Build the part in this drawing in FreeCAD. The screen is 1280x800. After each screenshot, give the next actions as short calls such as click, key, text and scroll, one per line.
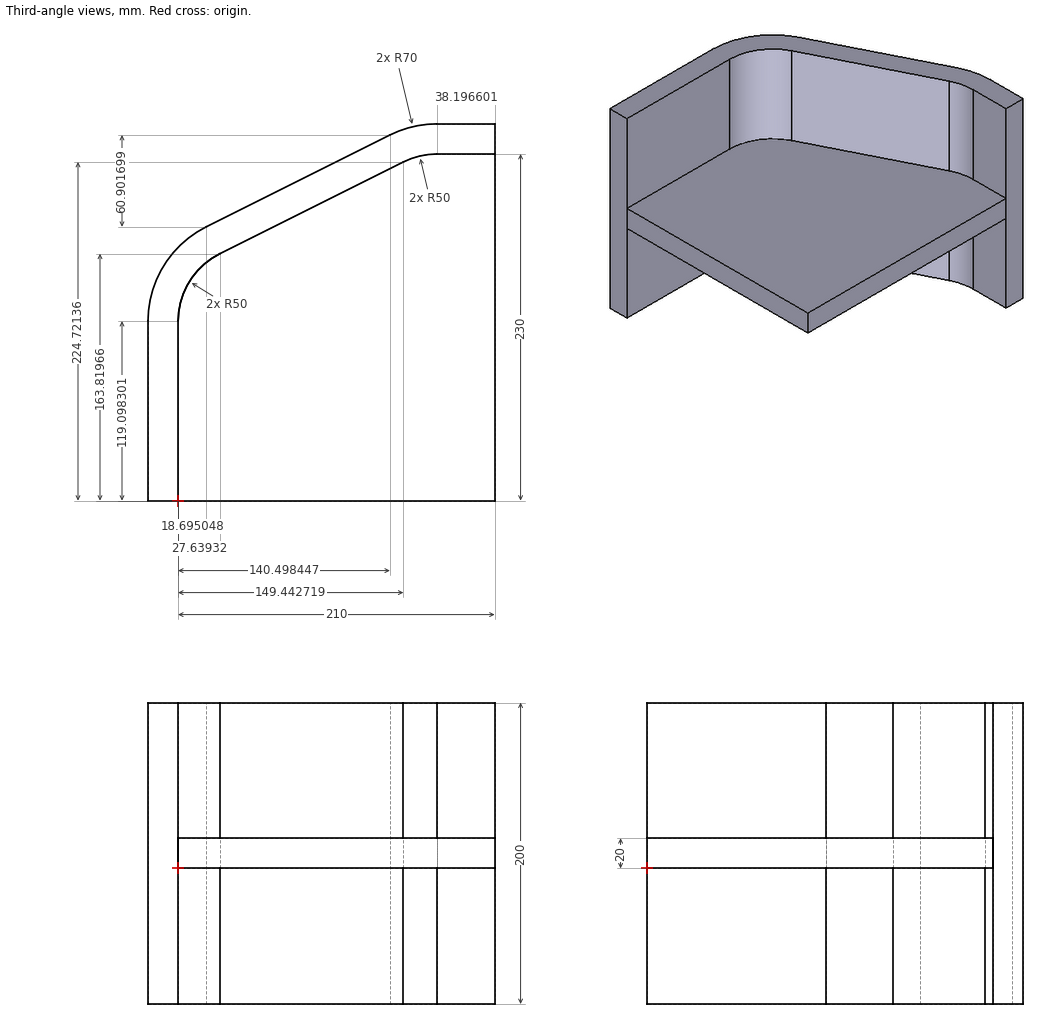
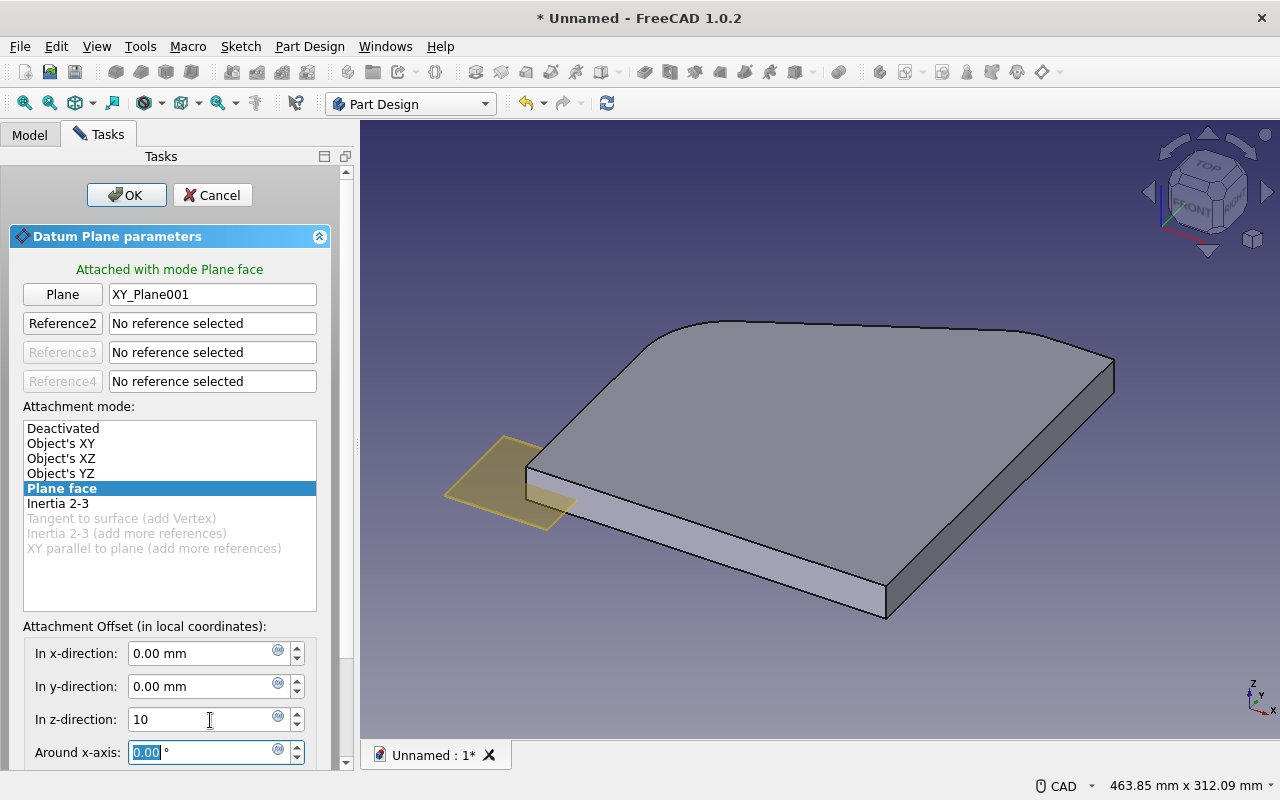
click(127, 195)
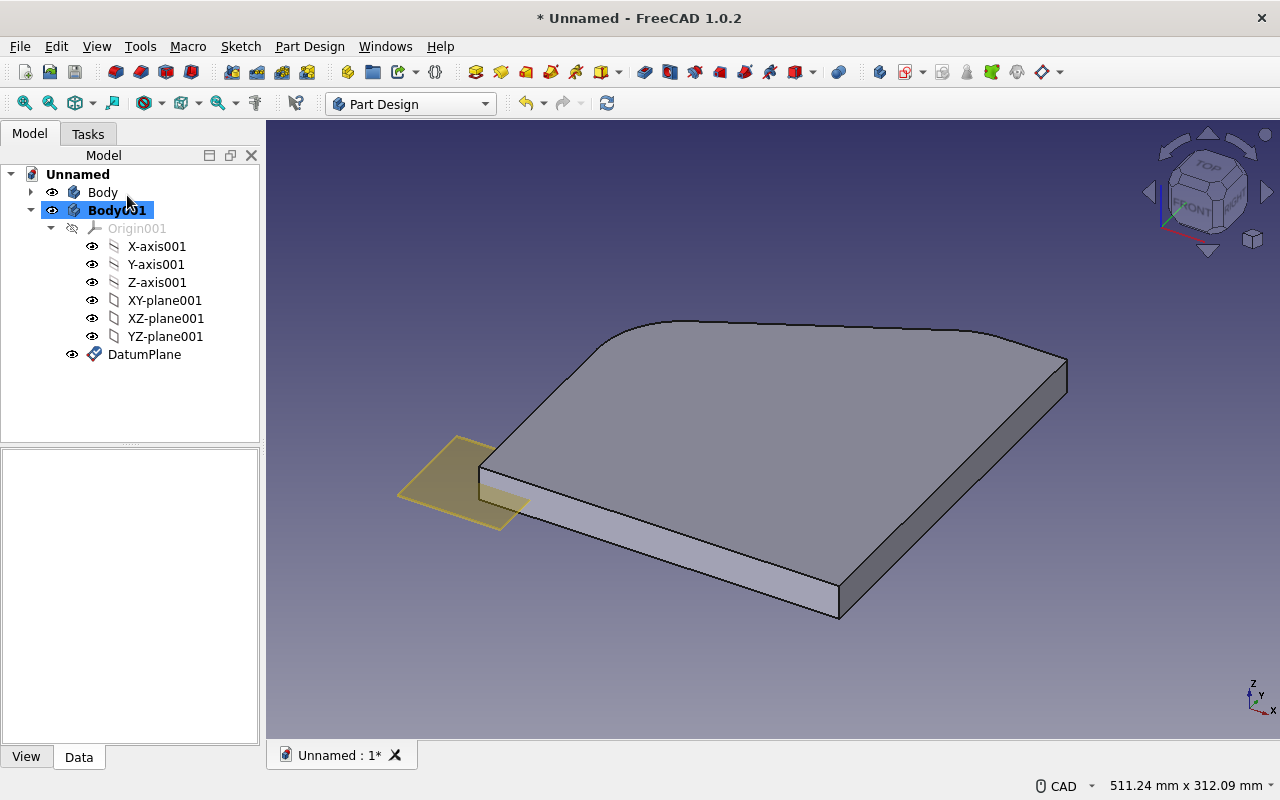
click(117, 354)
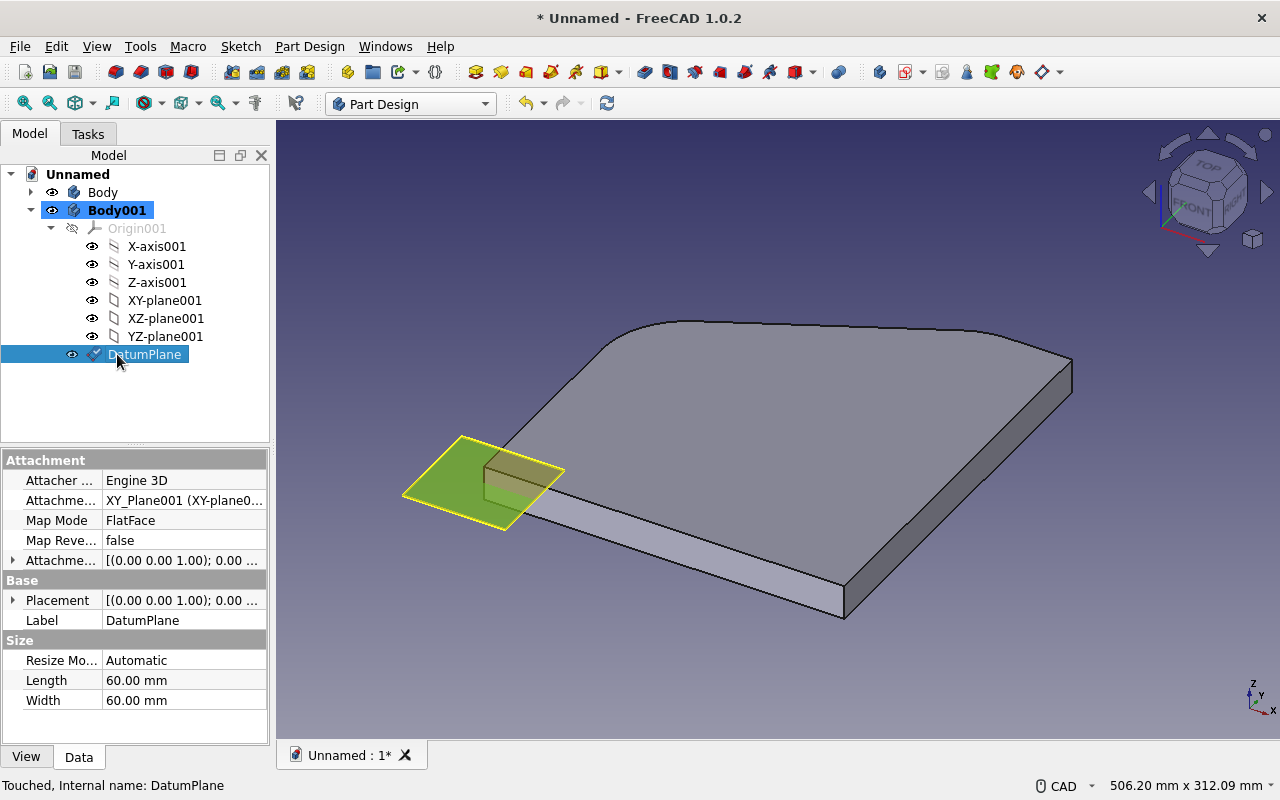
click(904, 72)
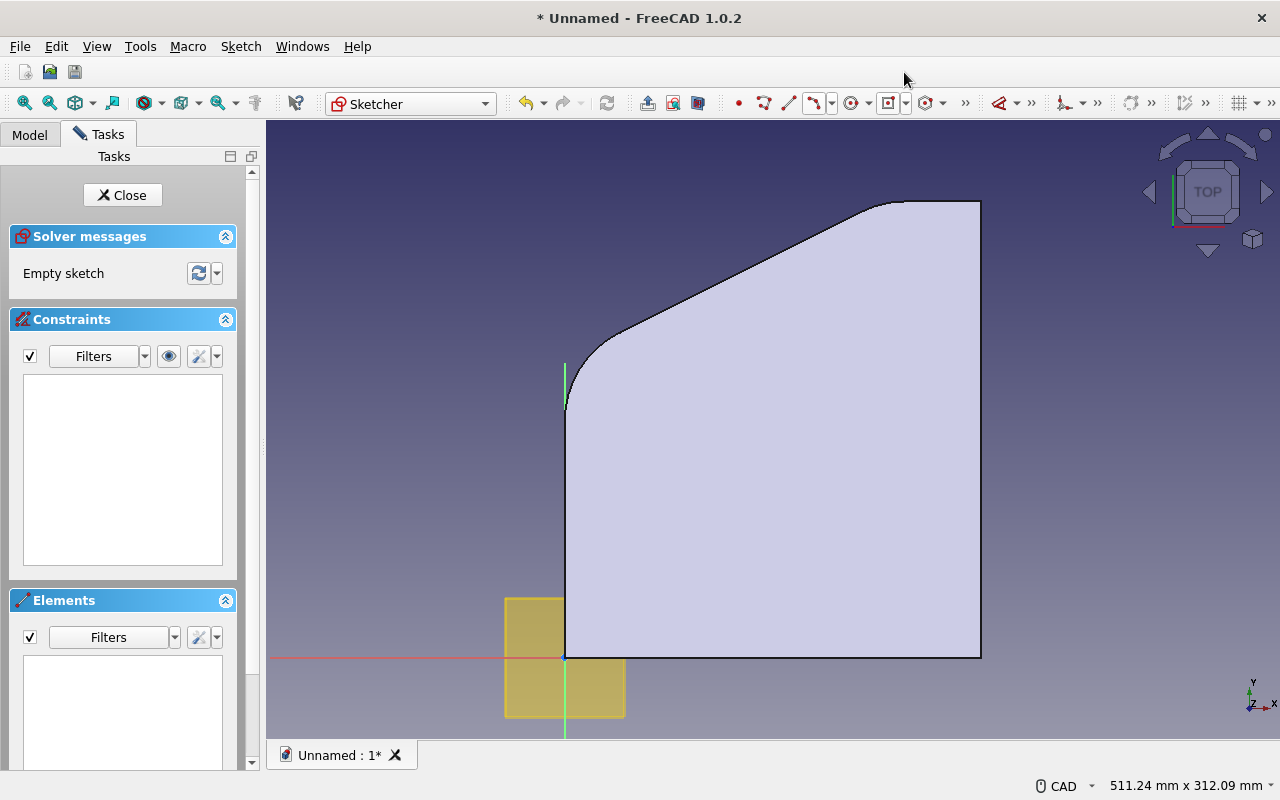
scroll(485, 519, down, 1)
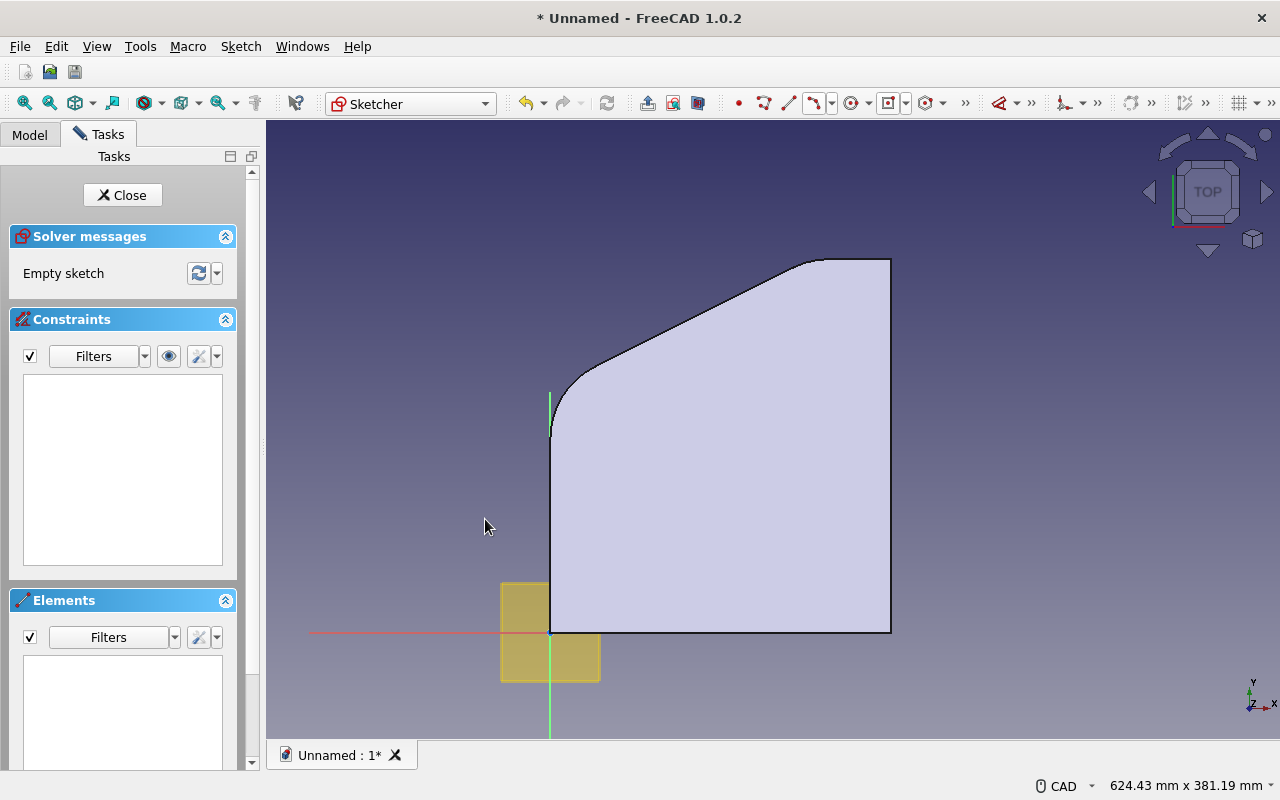
click(789, 104)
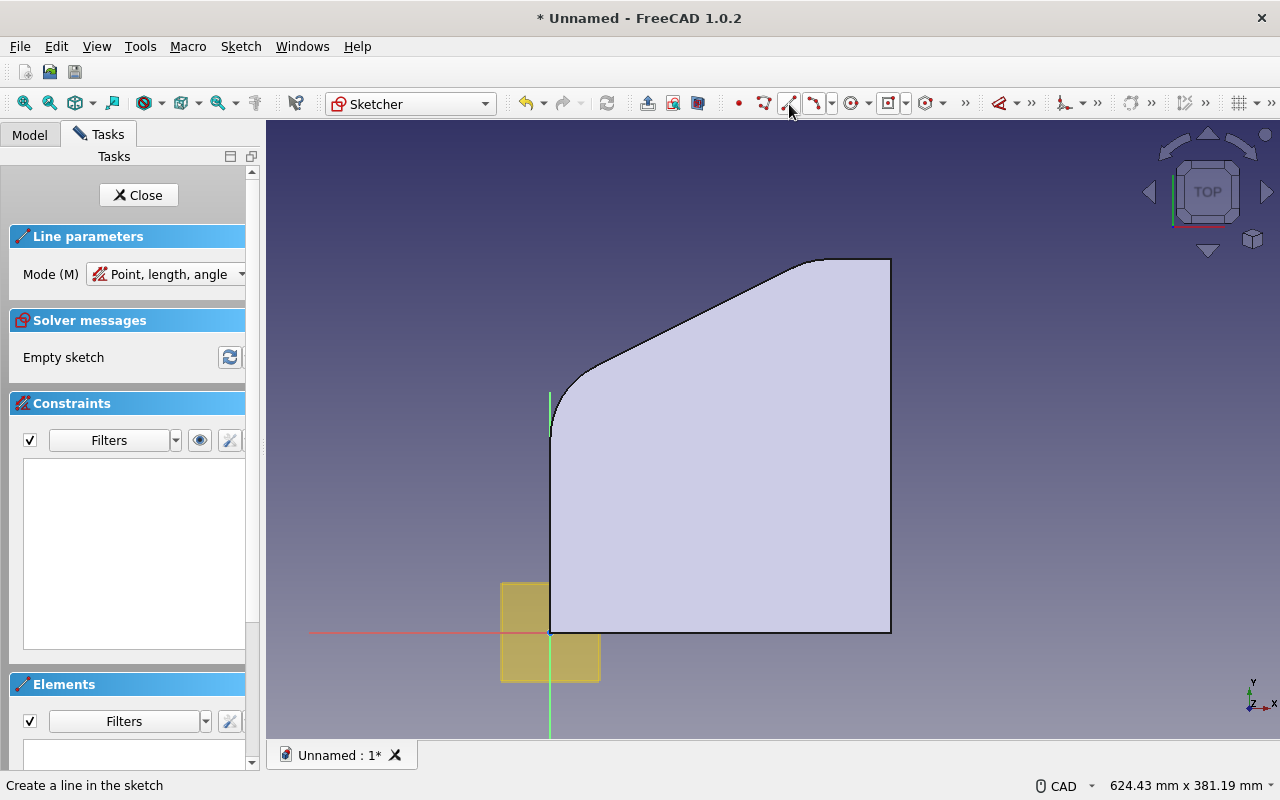
click(778, 239)
click(581, 338)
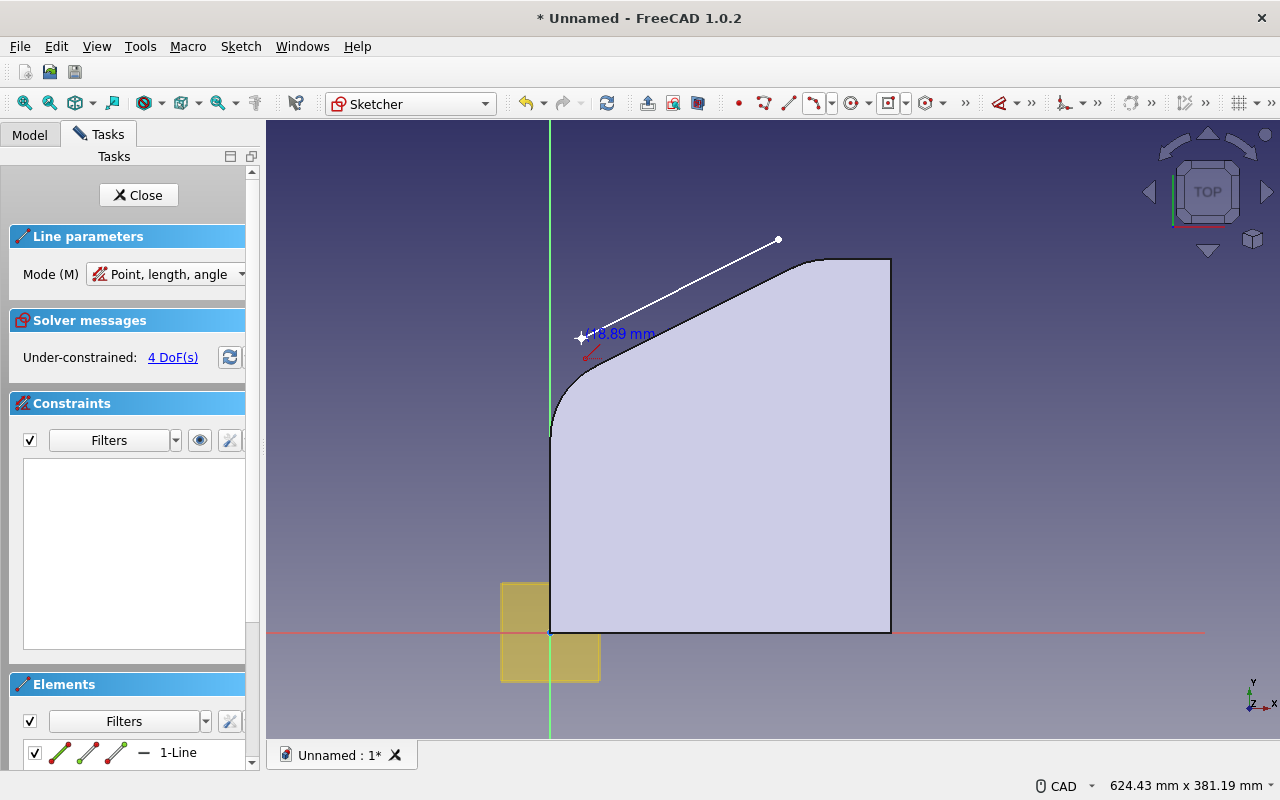
click(764, 104)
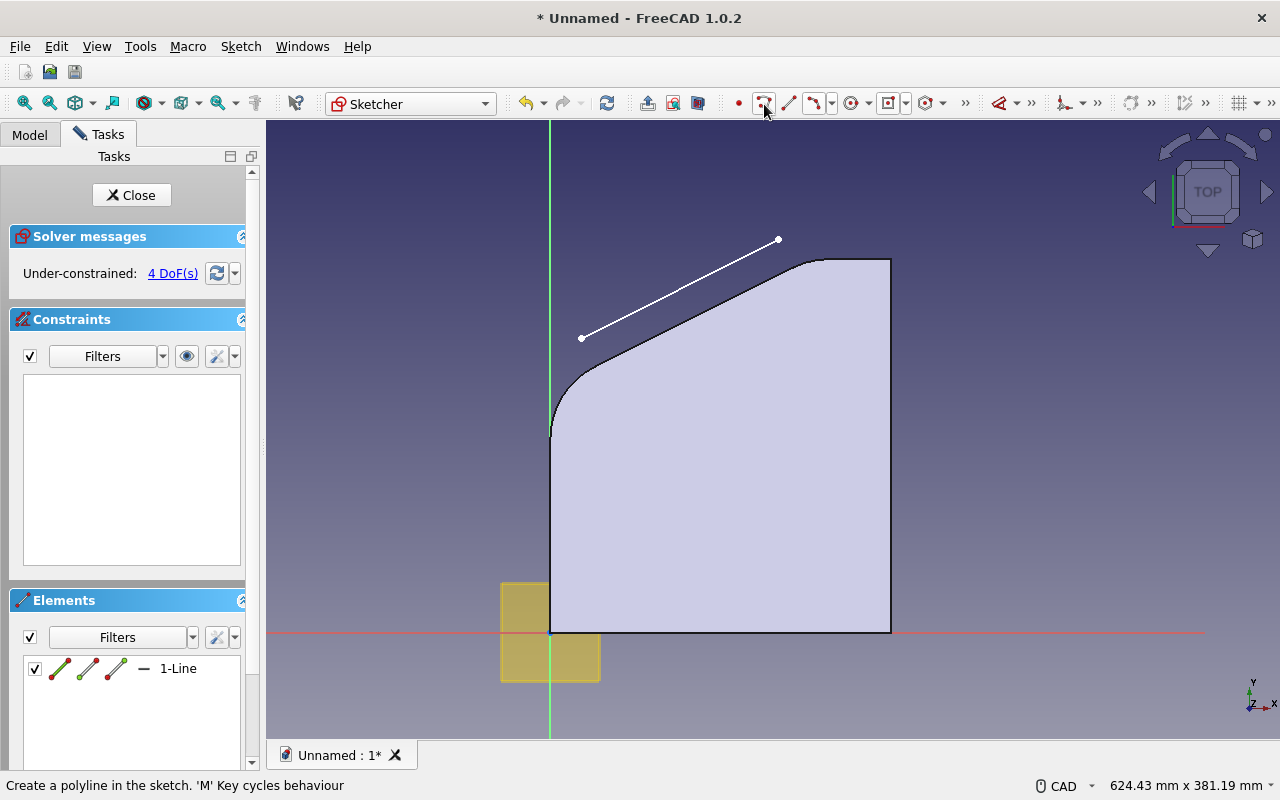
click(518, 439)
click(518, 633)
click(550, 633)
click(559, 439)
right_click(559, 439)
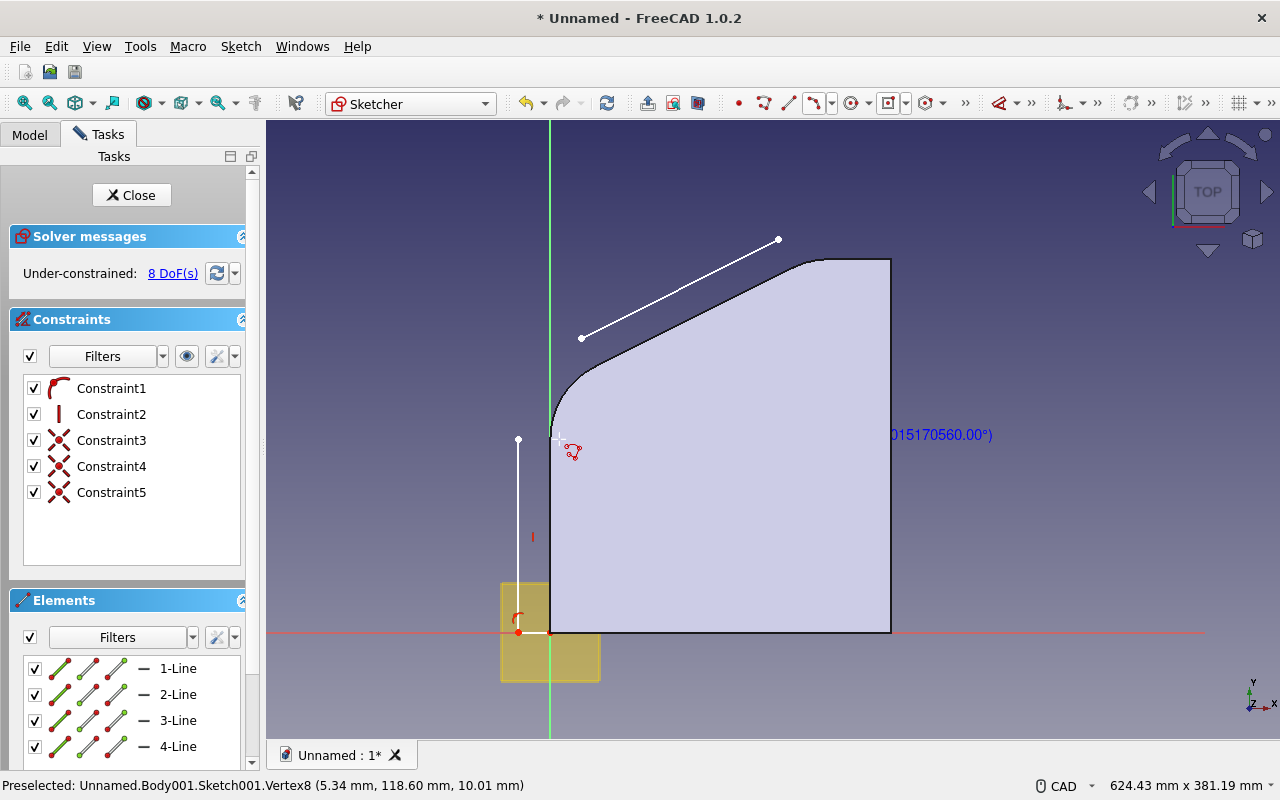
click(789, 104)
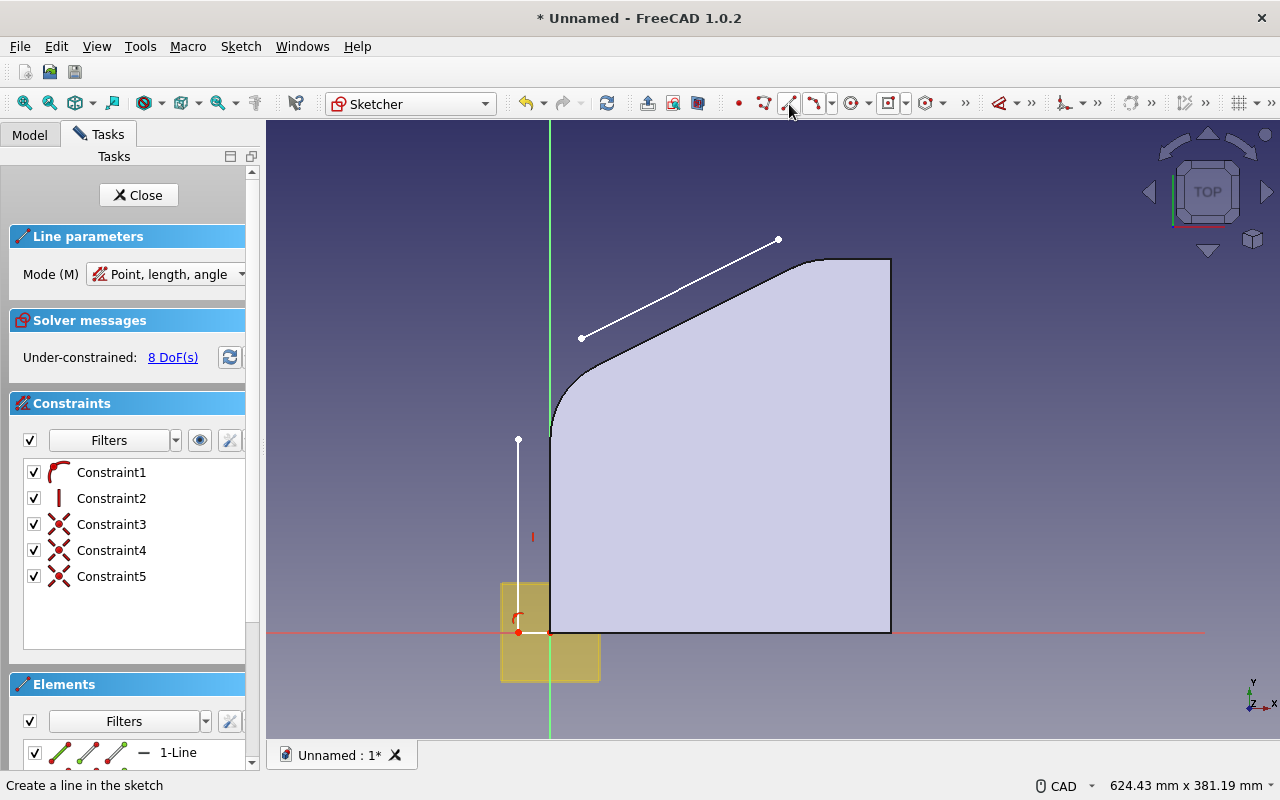
click(595, 367)
click(793, 268)